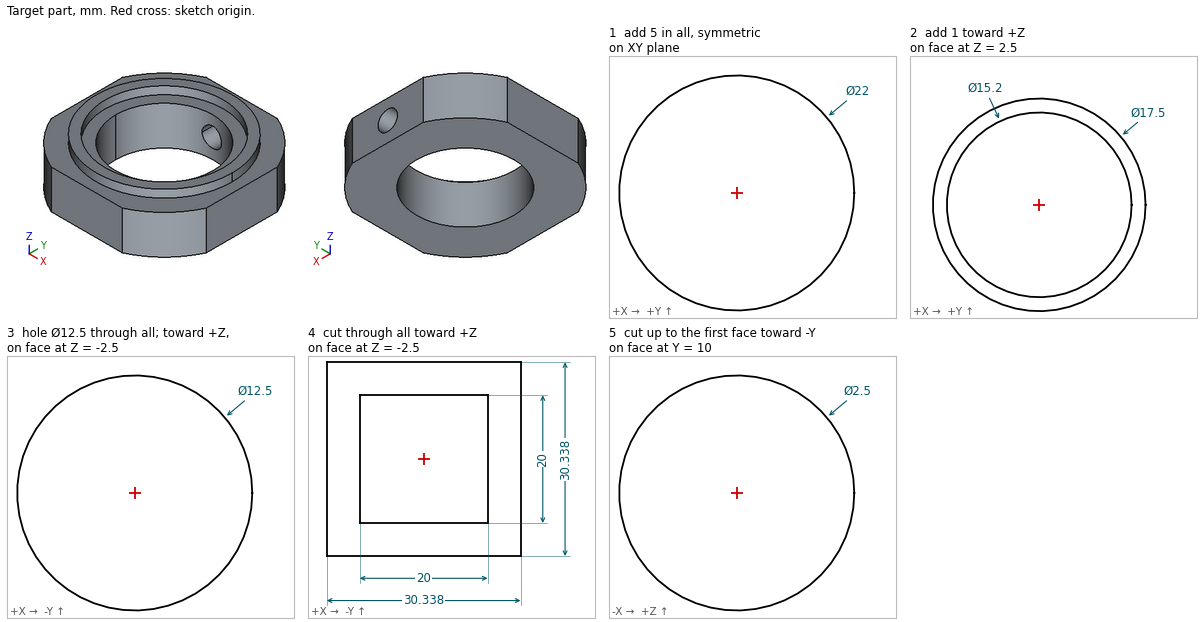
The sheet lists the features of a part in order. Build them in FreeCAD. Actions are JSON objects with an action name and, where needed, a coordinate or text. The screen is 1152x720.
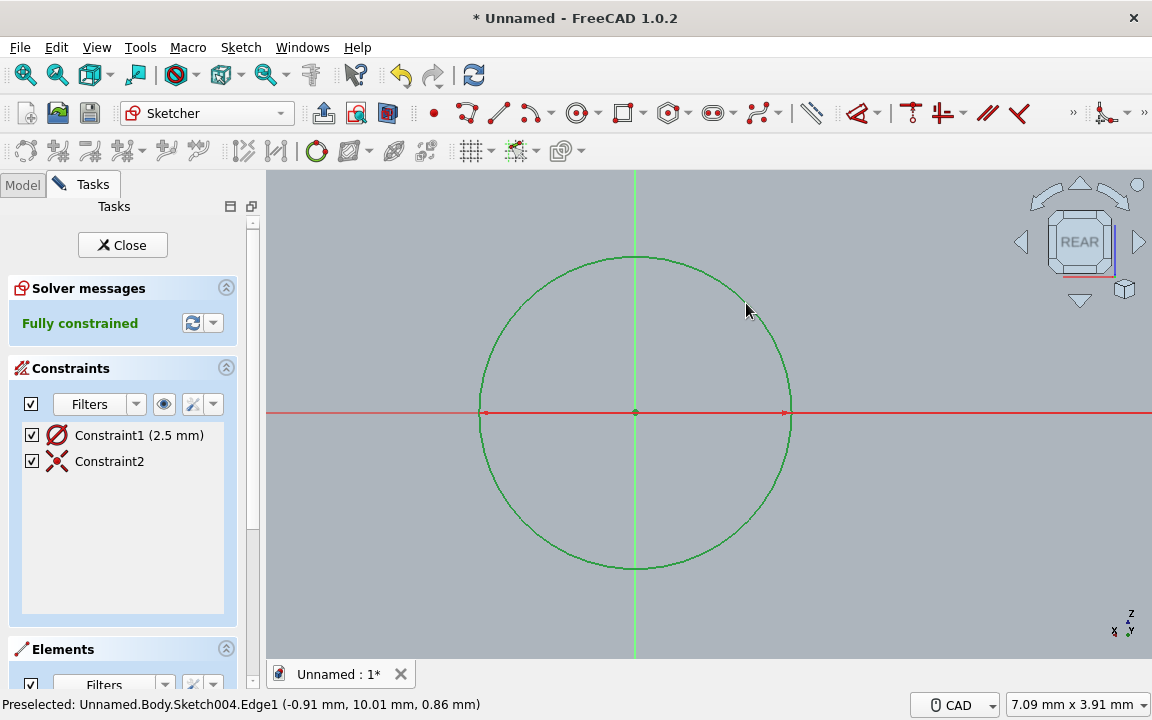
{"action": "left_click", "coordinate": [123, 245]}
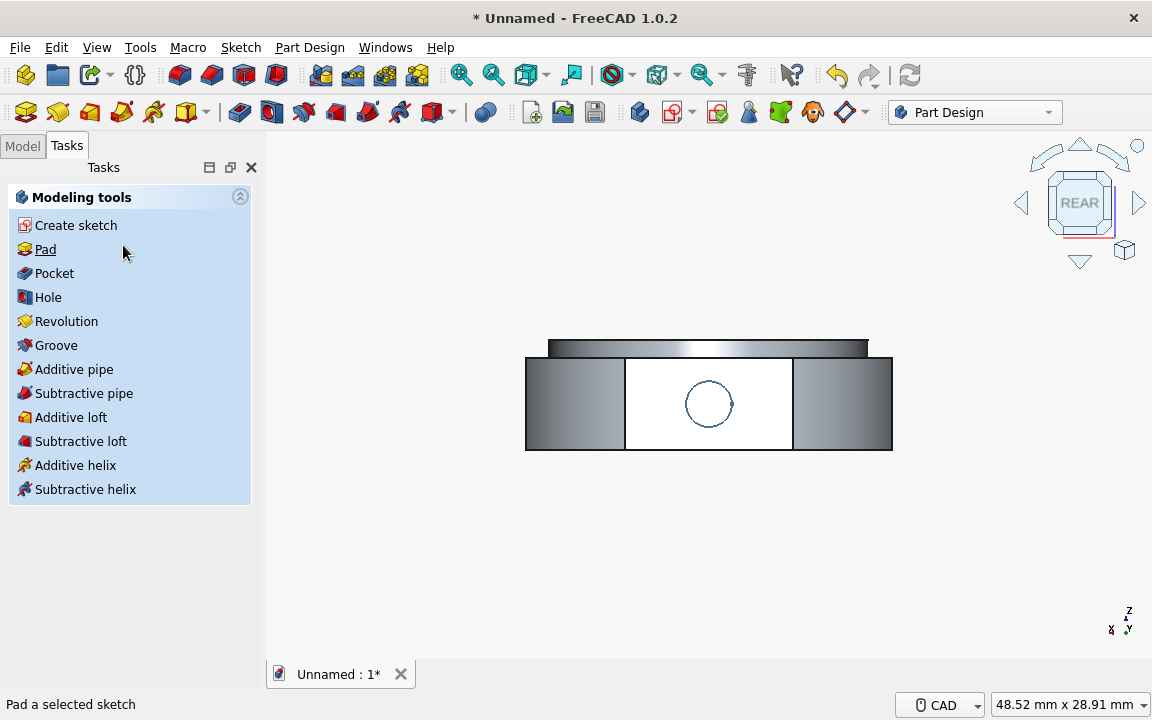
{"action": "left_click", "coordinate": [240, 112]}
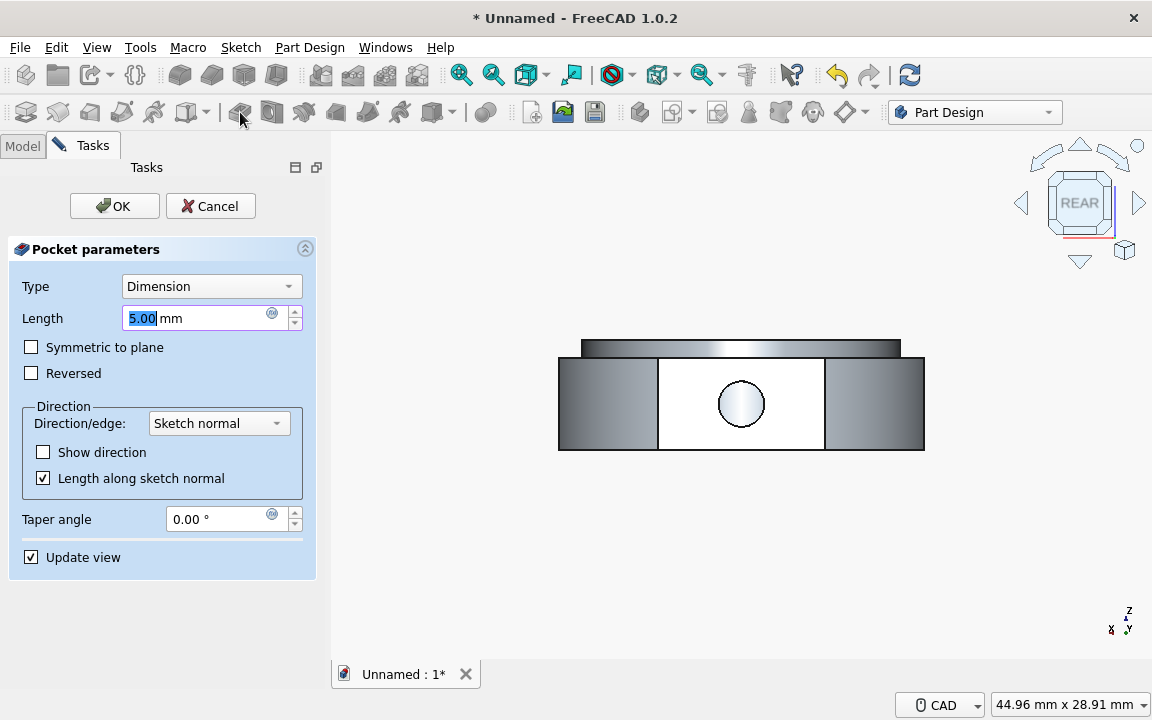
{"action": "left_click", "coordinate": [212, 286]}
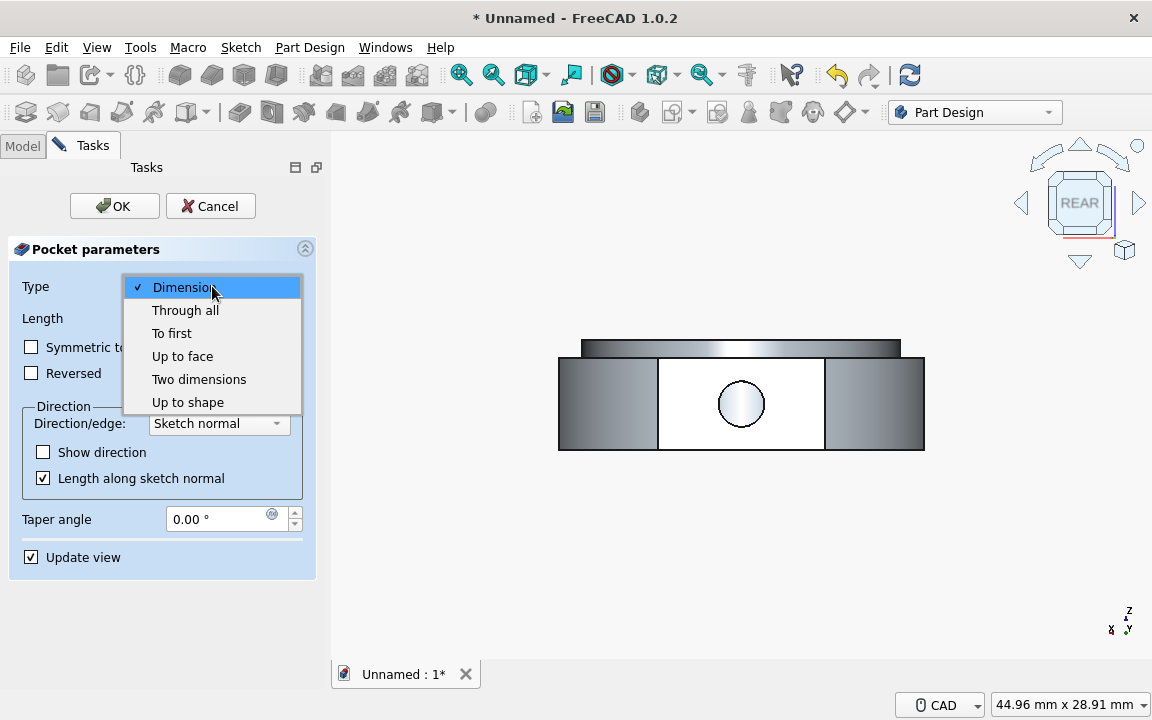
{"action": "left_click", "coordinate": [212, 334]}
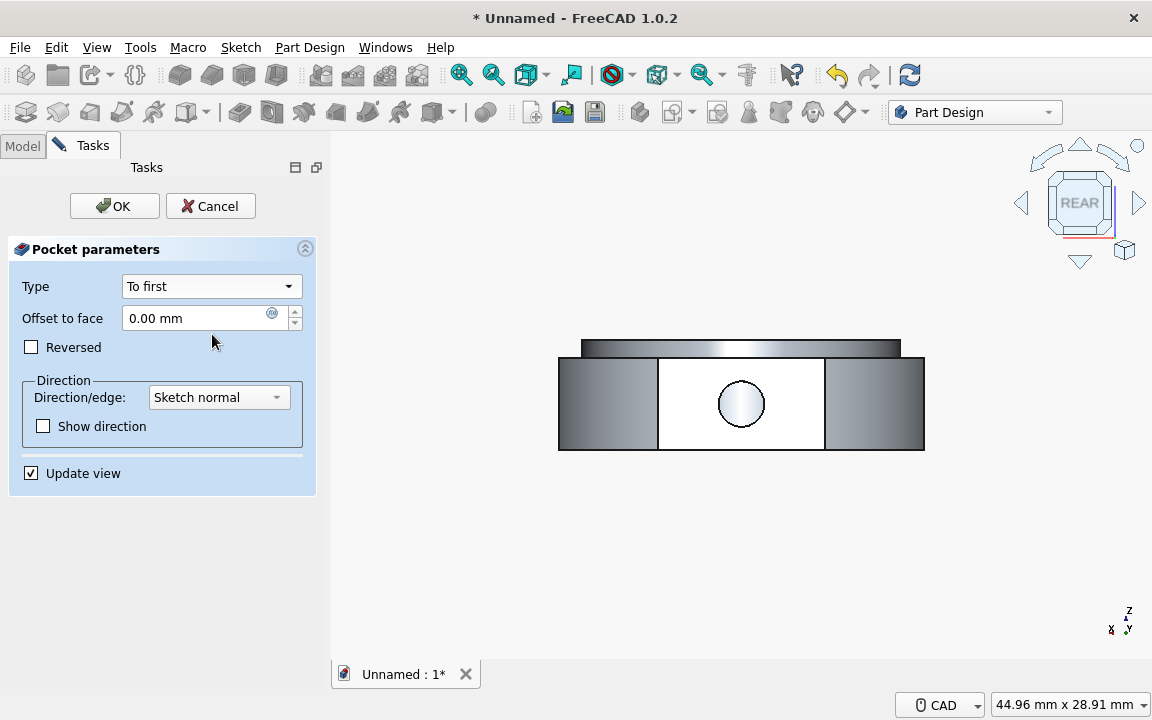
{"action": "left_click", "coordinate": [115, 206]}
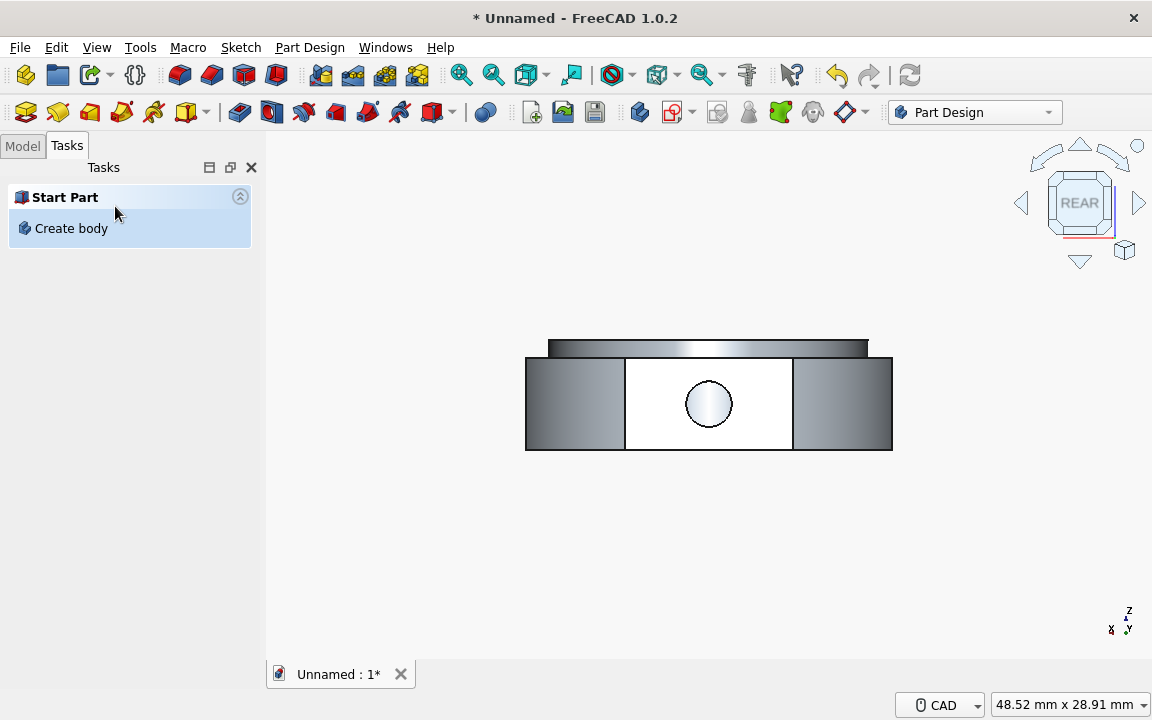
{"action": "key", "text": "0"}